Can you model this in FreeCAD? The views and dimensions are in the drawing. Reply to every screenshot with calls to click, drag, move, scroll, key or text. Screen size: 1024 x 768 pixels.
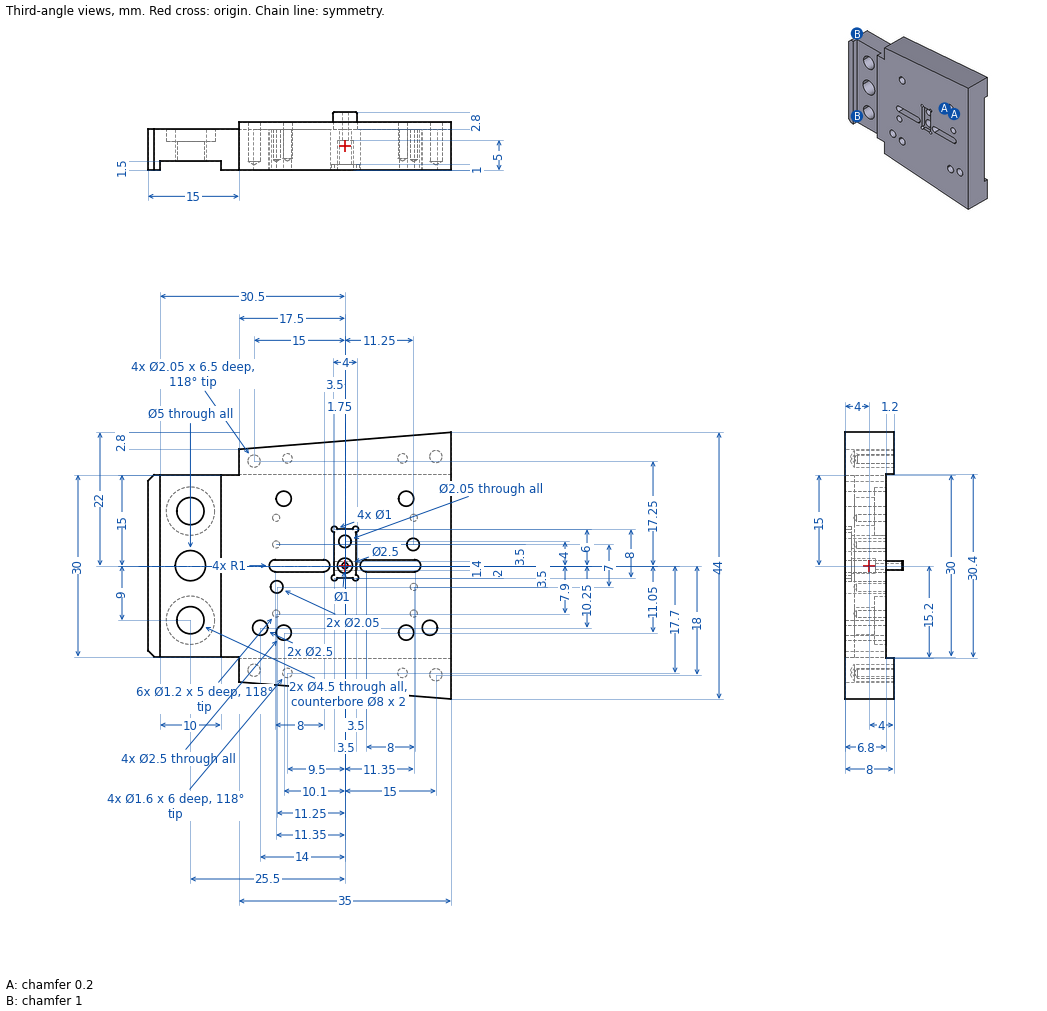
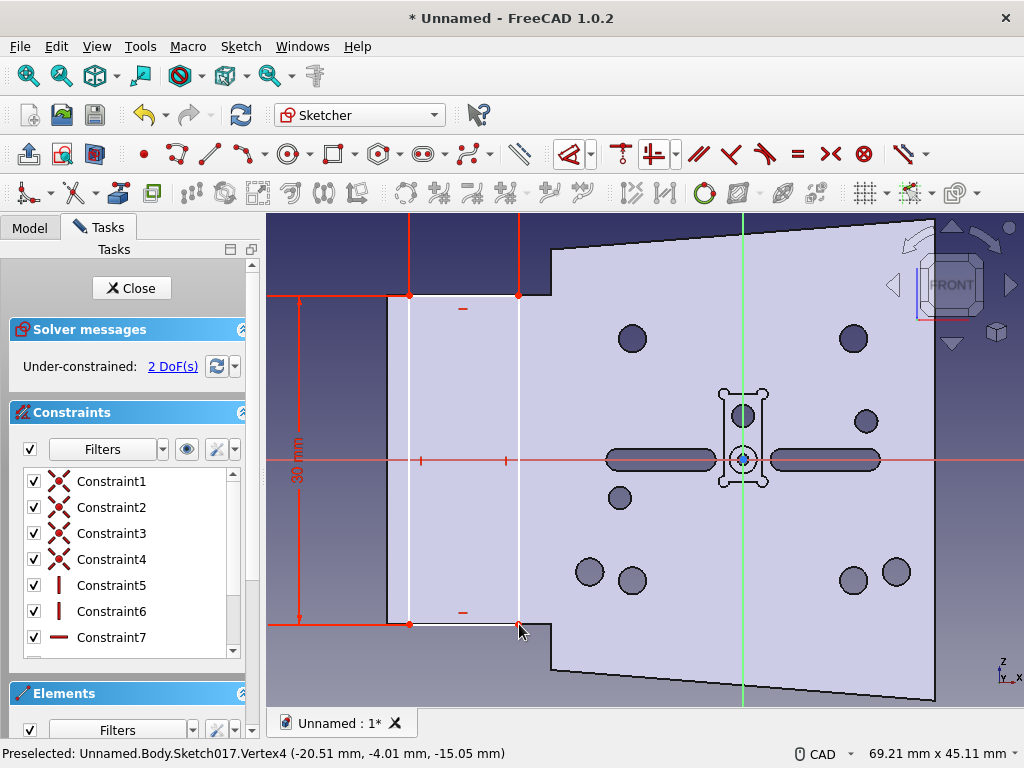
click(409, 296)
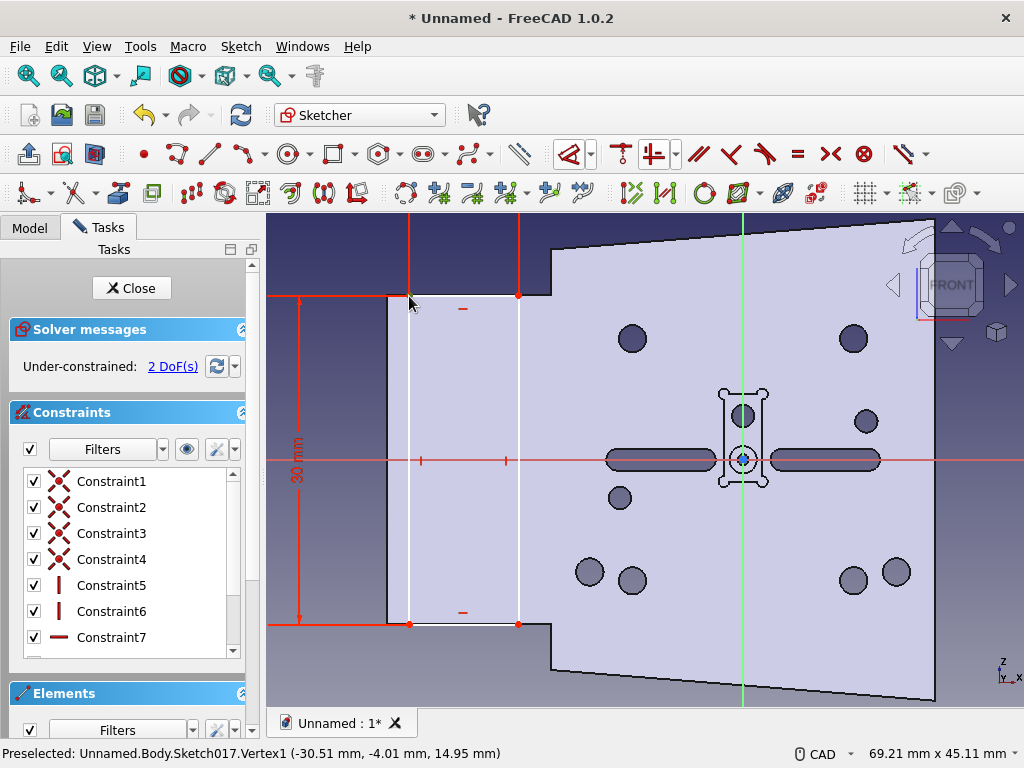
key(i)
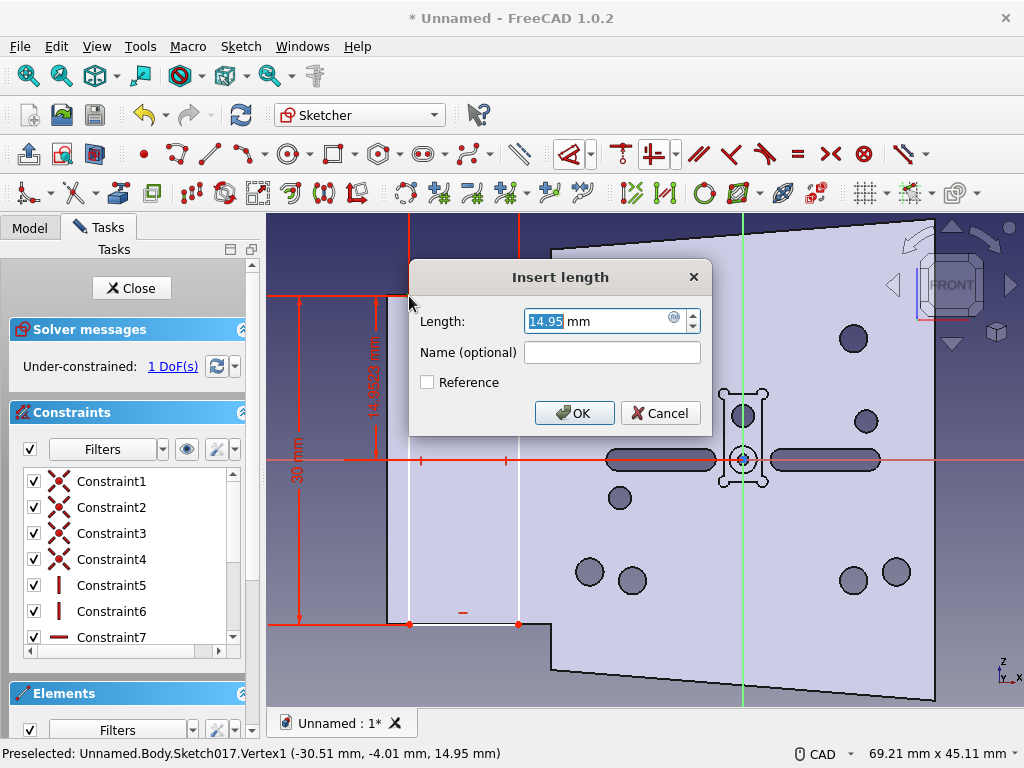
text(15)
key(Return)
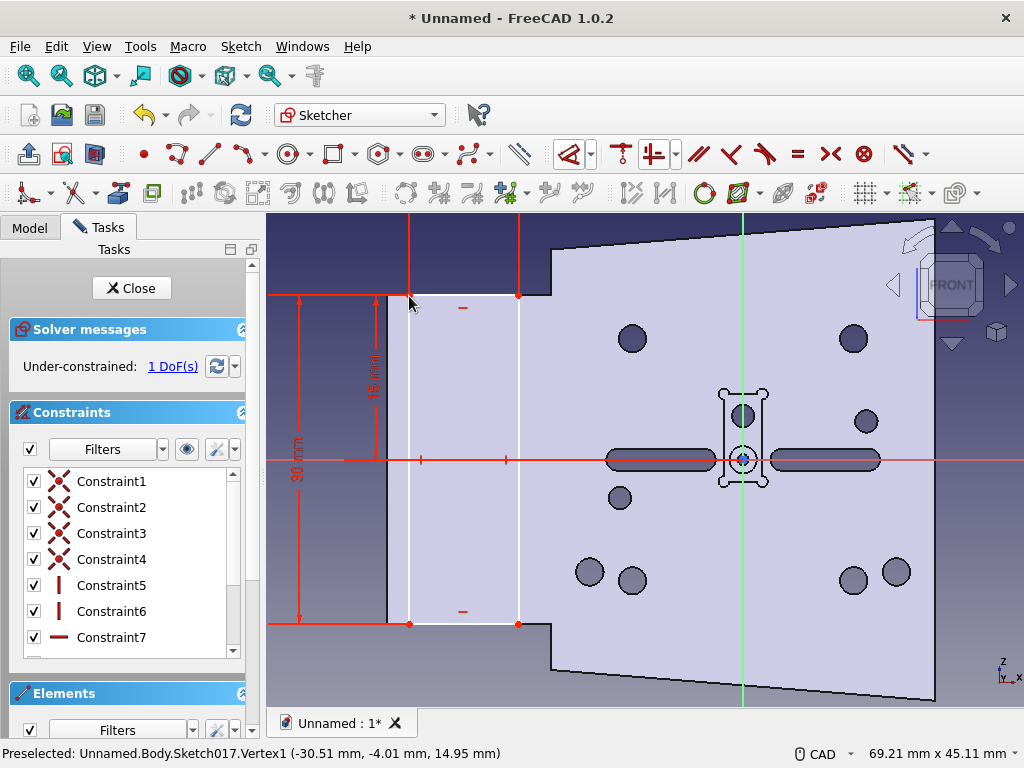
click(409, 295)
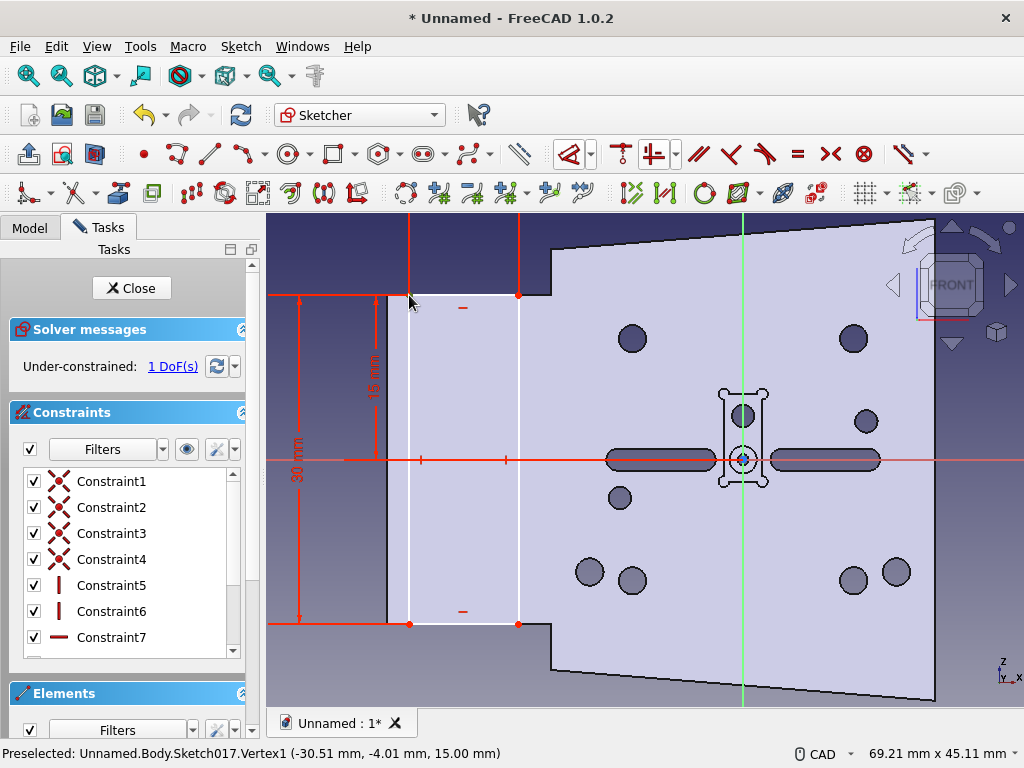
key(l)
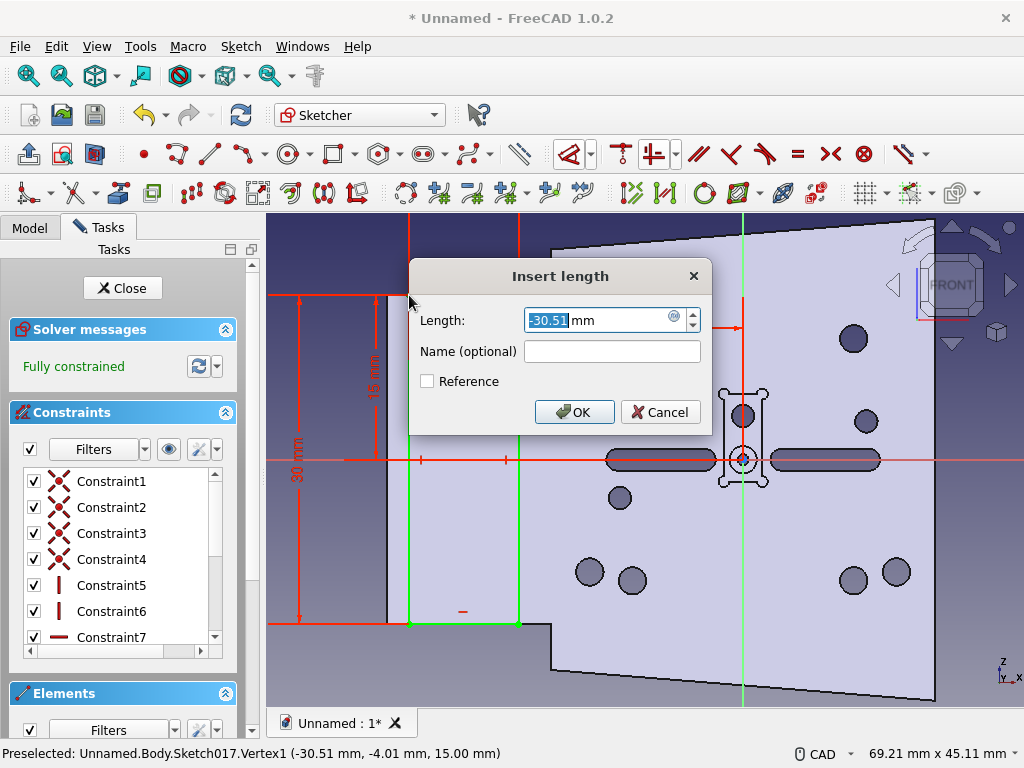
text(-30.5)
key(Return)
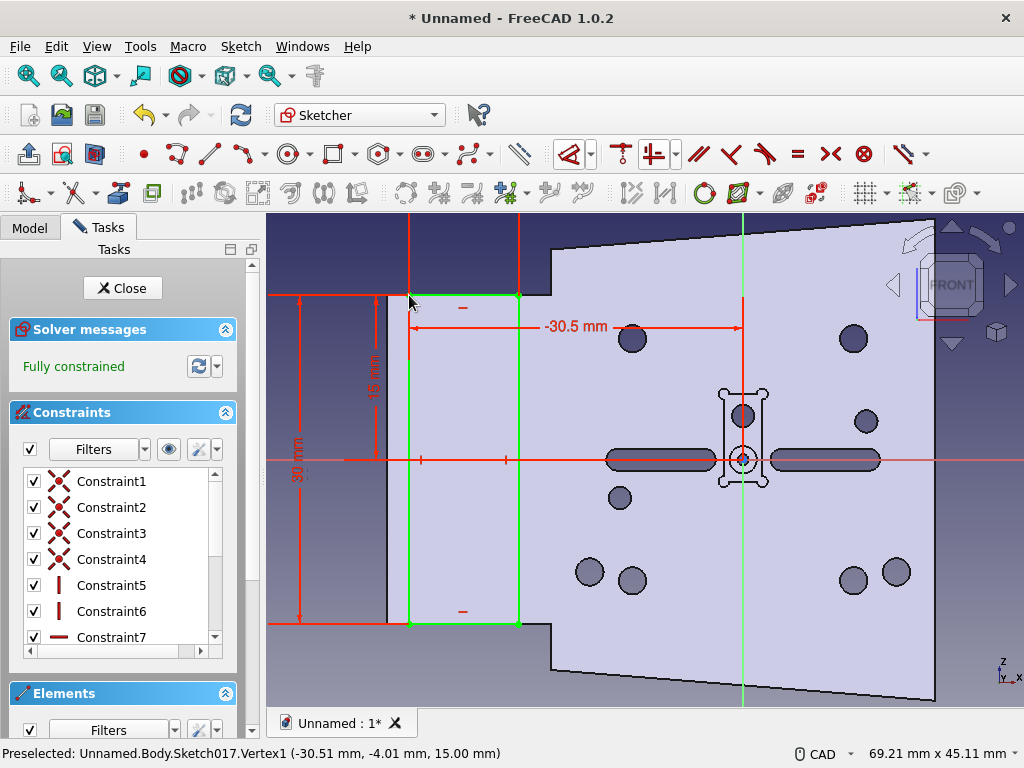
click(123, 288)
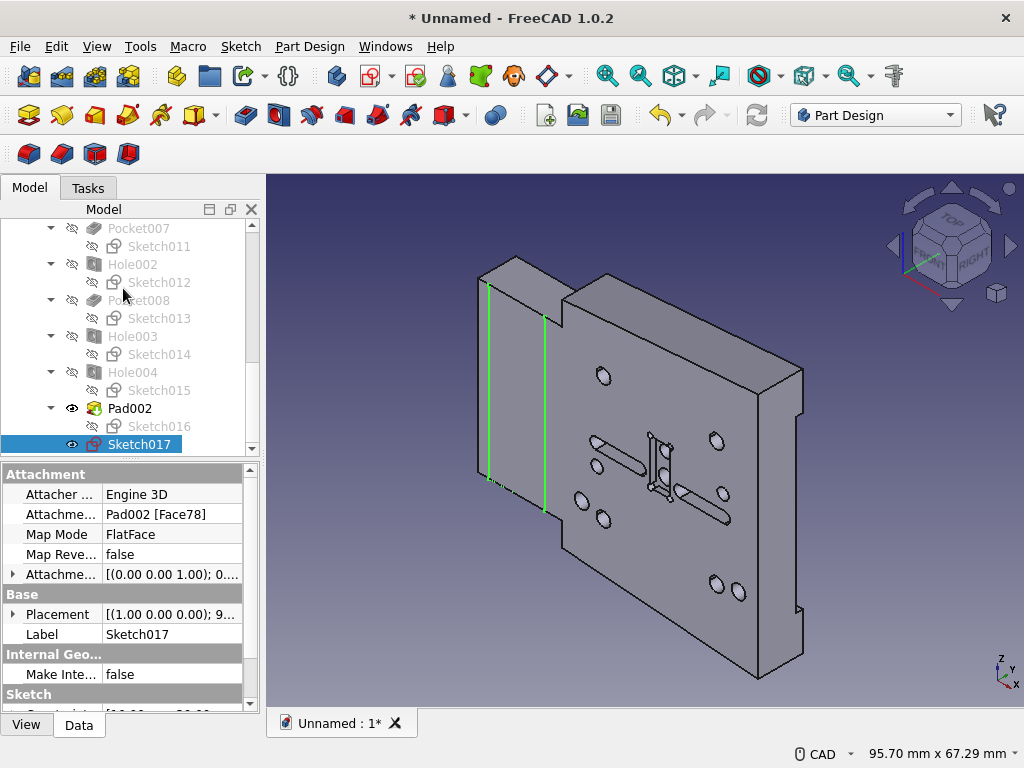
click(246, 116)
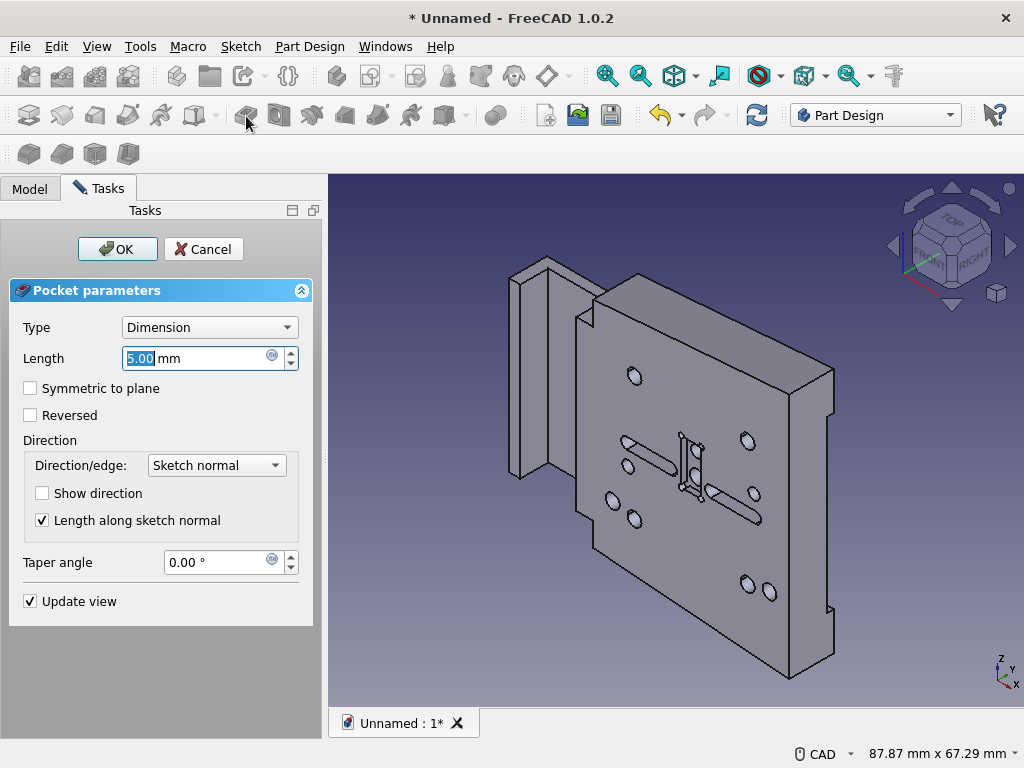
text(1.5)
key(Tab)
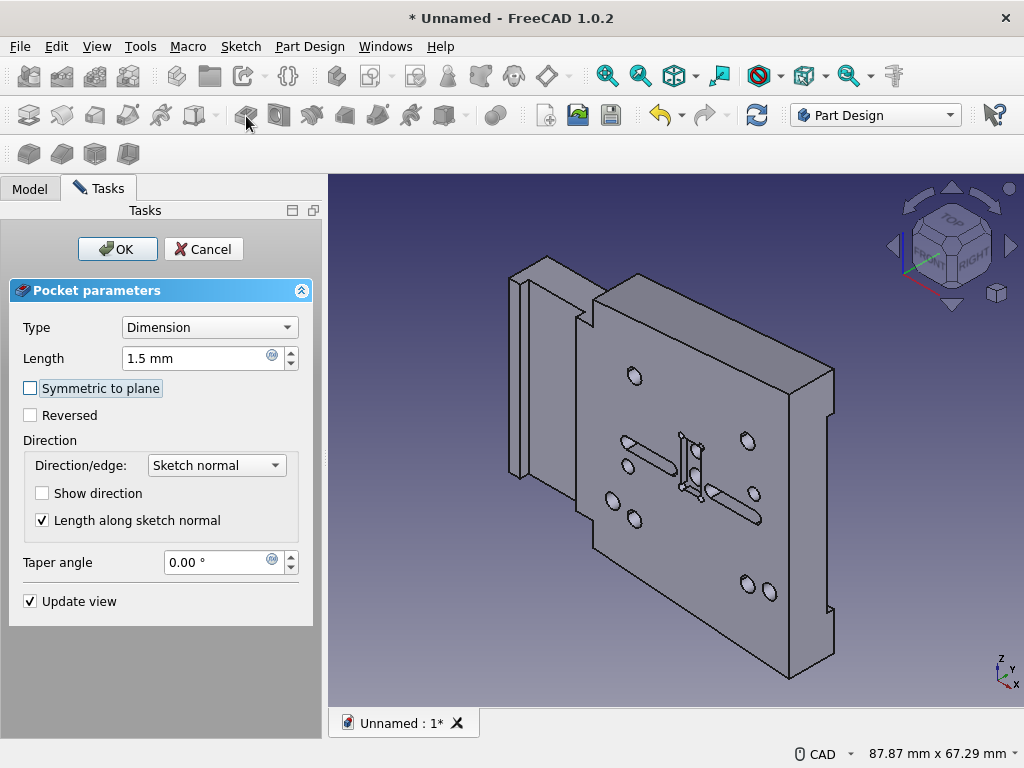
click(118, 249)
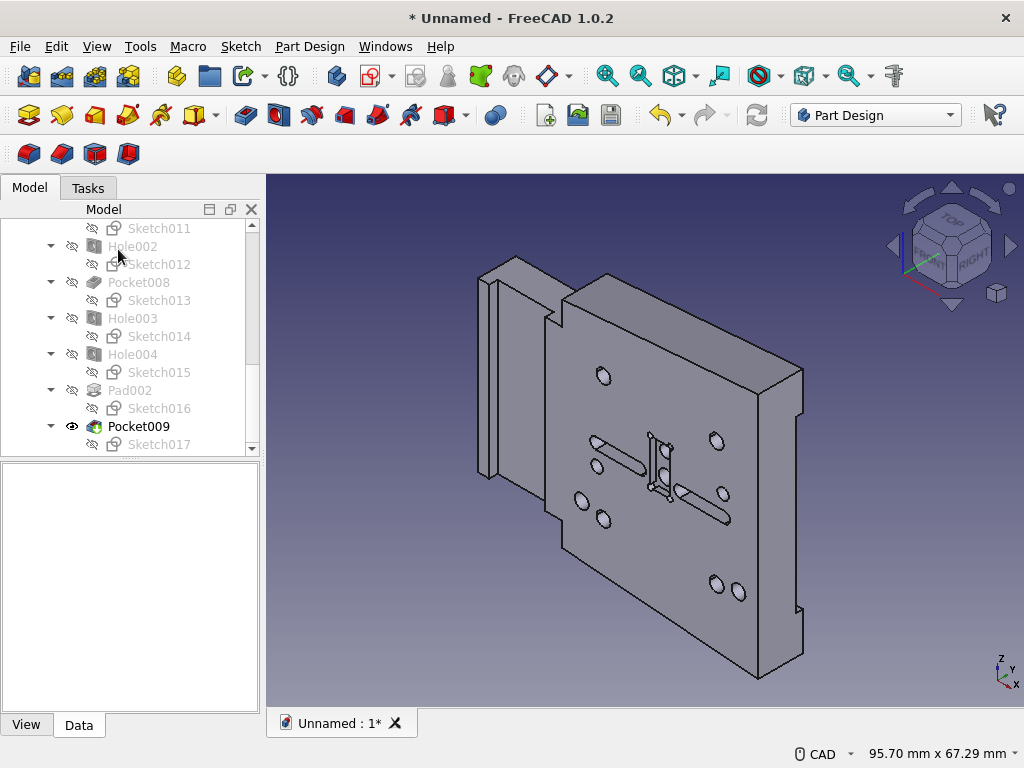
key(4)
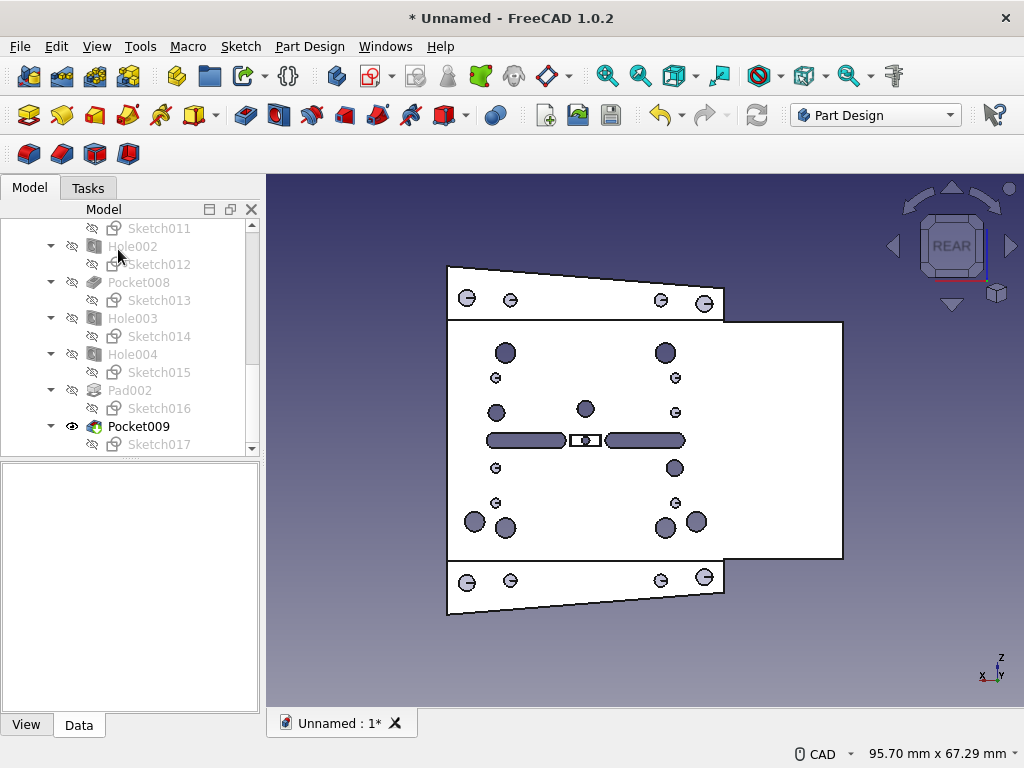
click(758, 405)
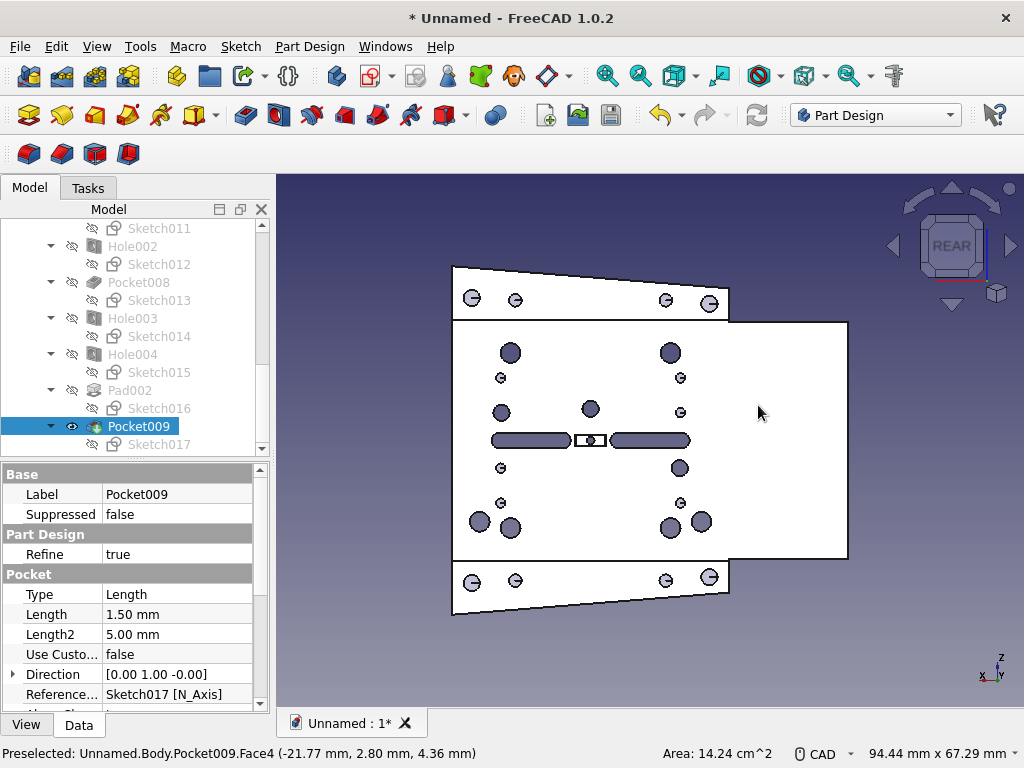
click(370, 76)